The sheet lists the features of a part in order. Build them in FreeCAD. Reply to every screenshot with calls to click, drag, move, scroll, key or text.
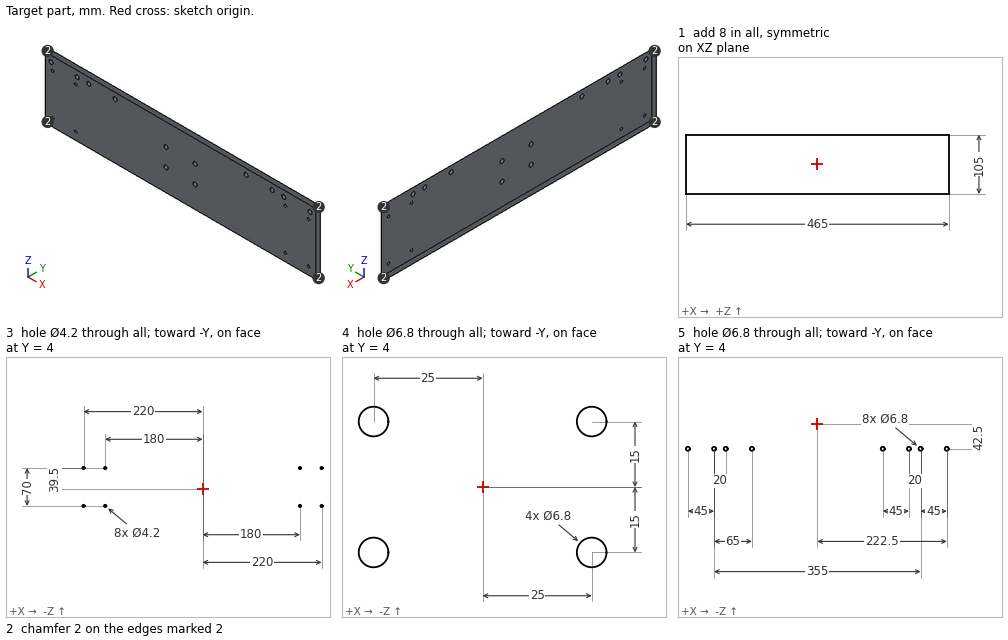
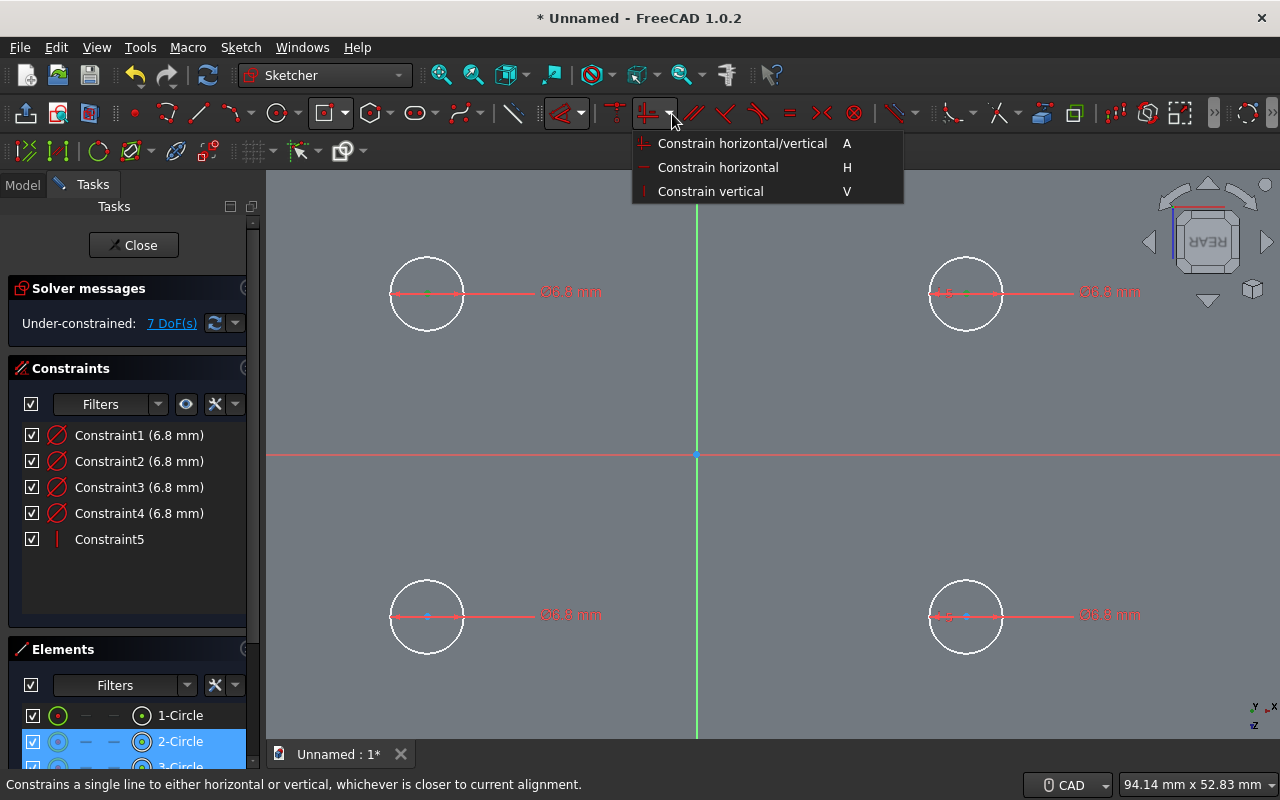
click(768, 167)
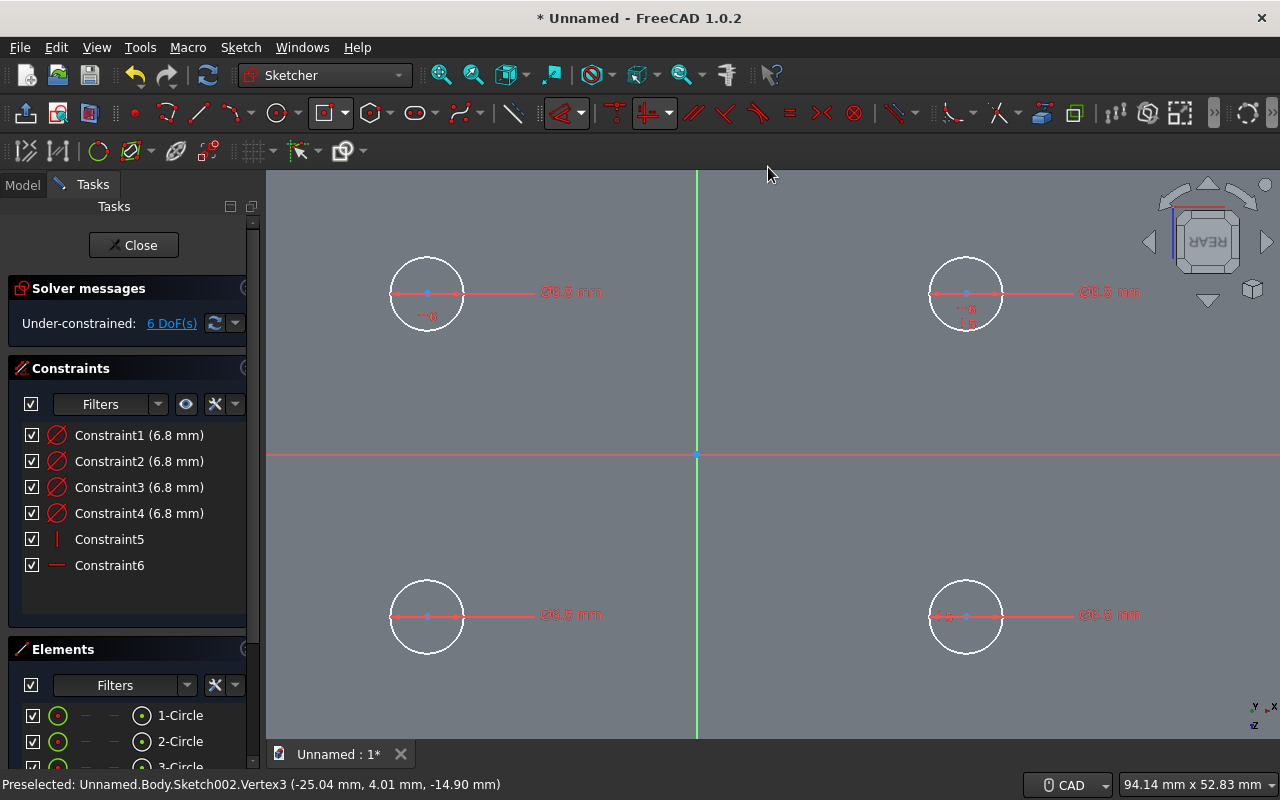
click(427, 294)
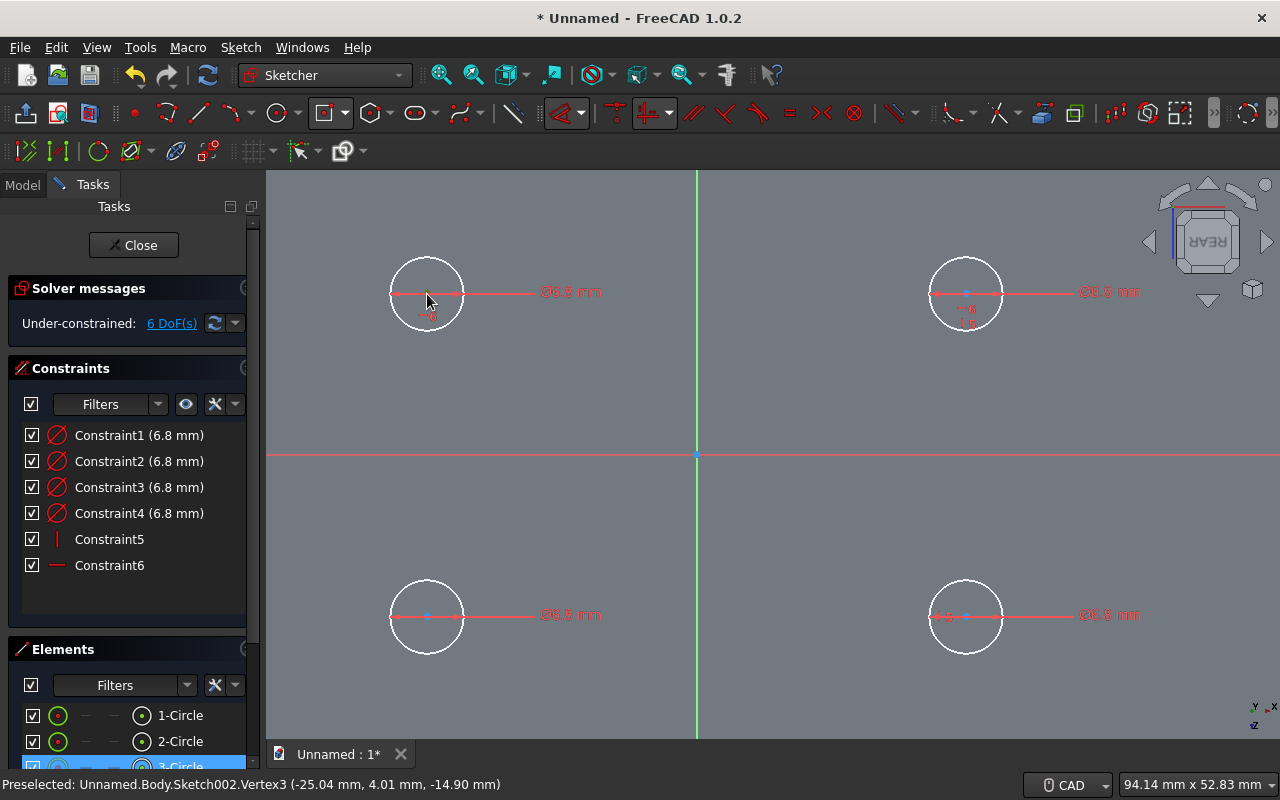
click(427, 617)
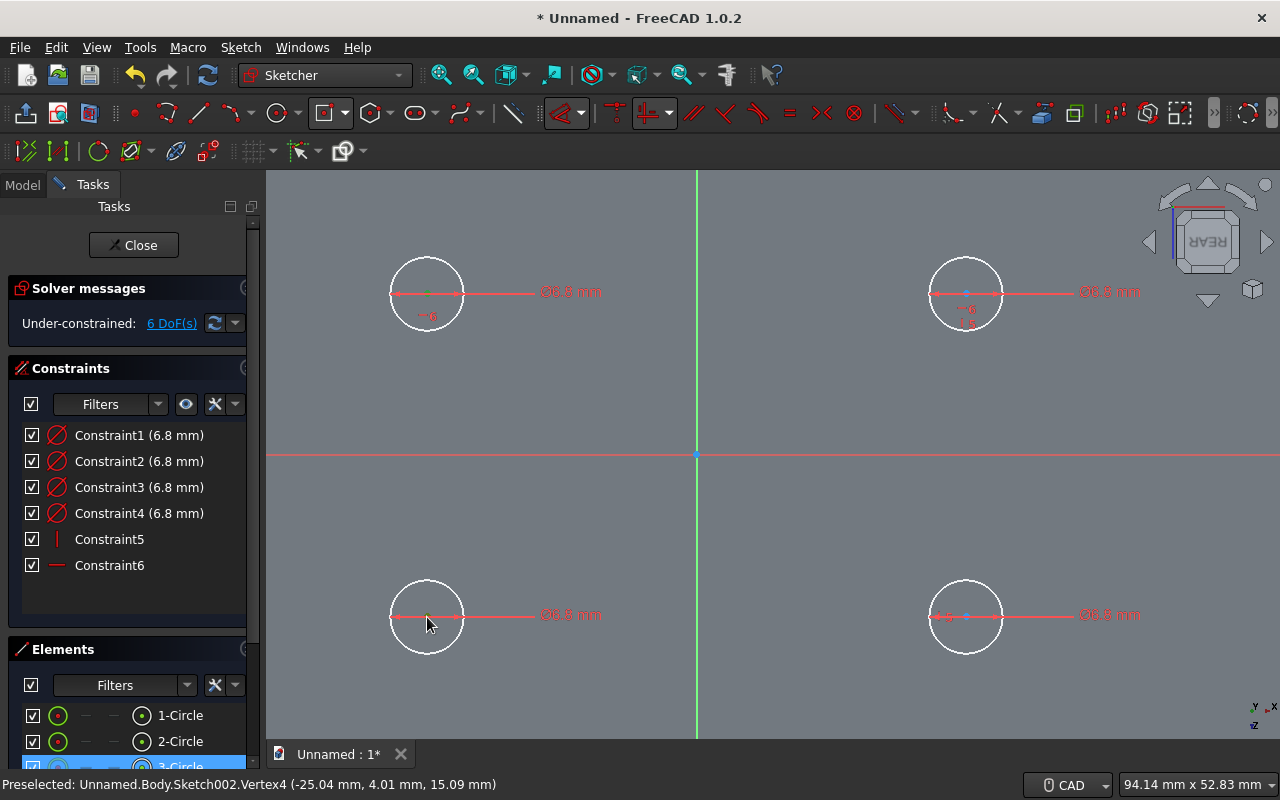
key(v)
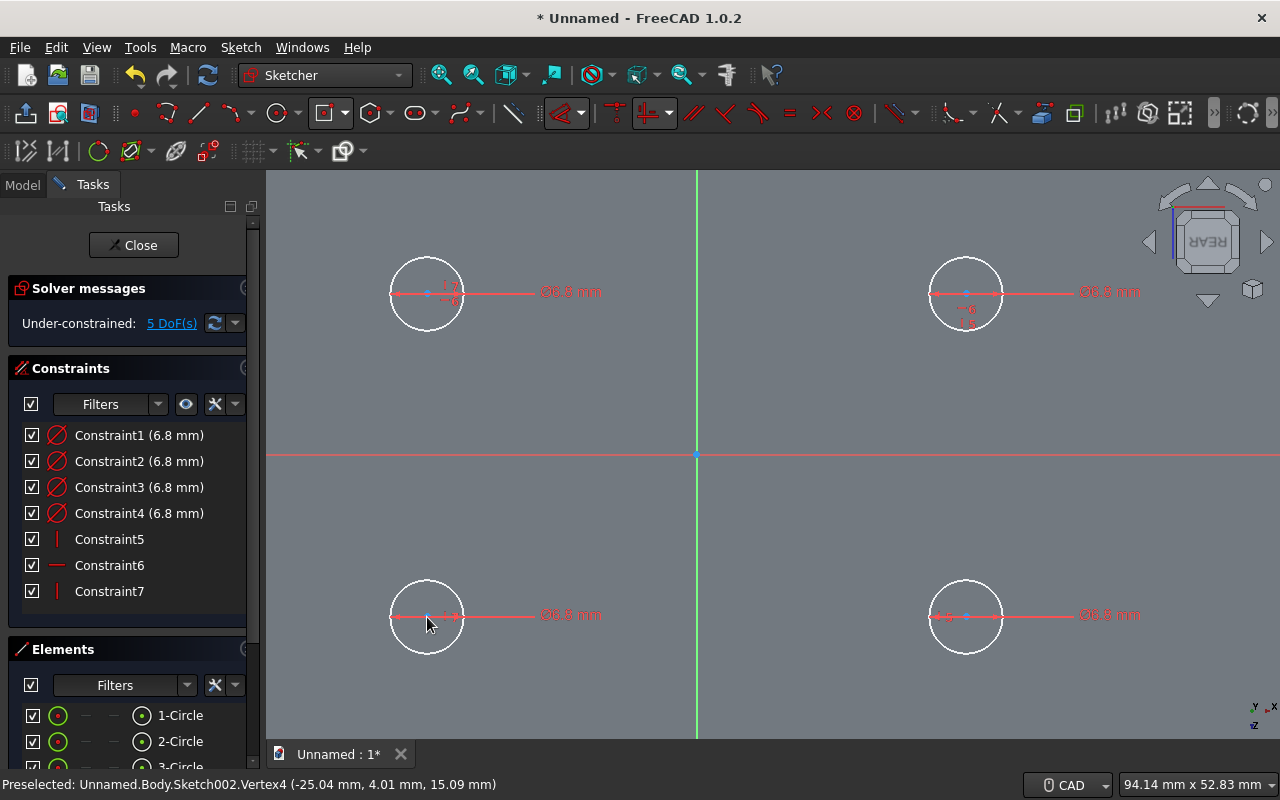
click(966, 617)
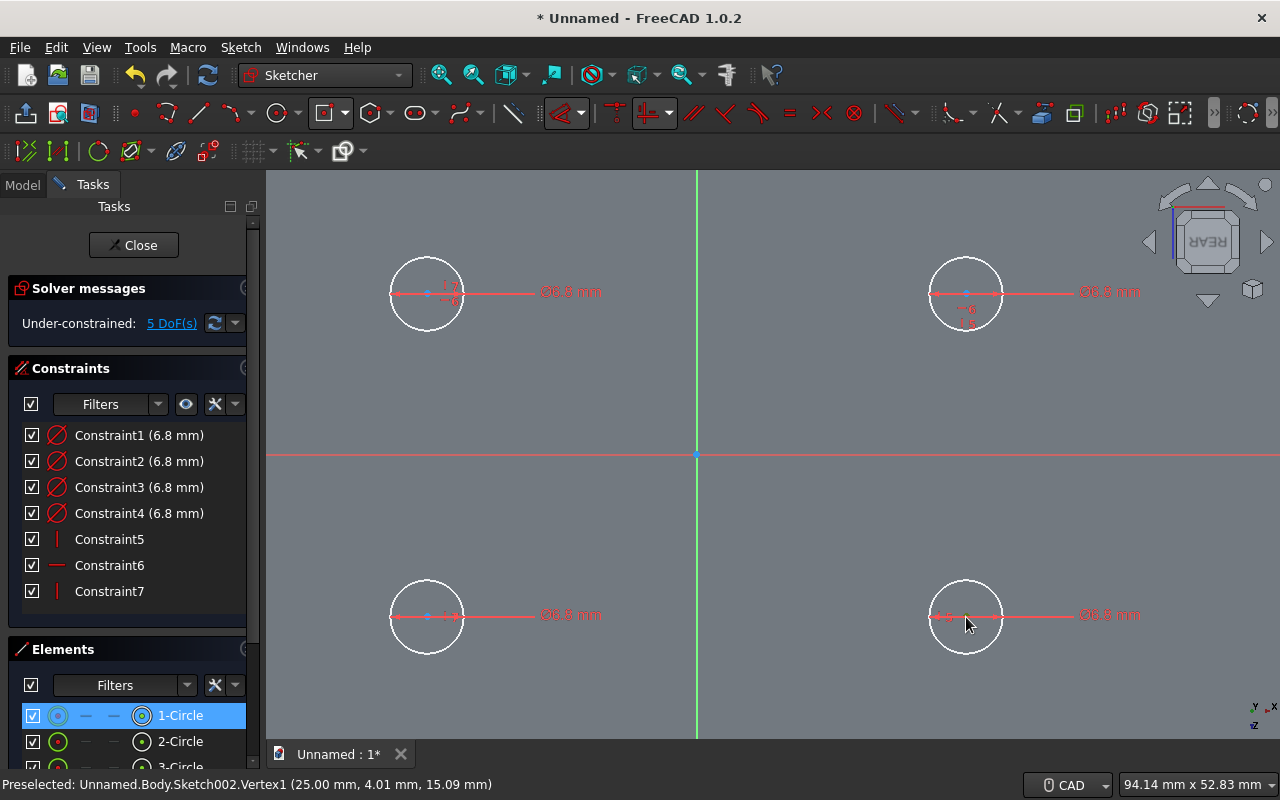
click(427, 617)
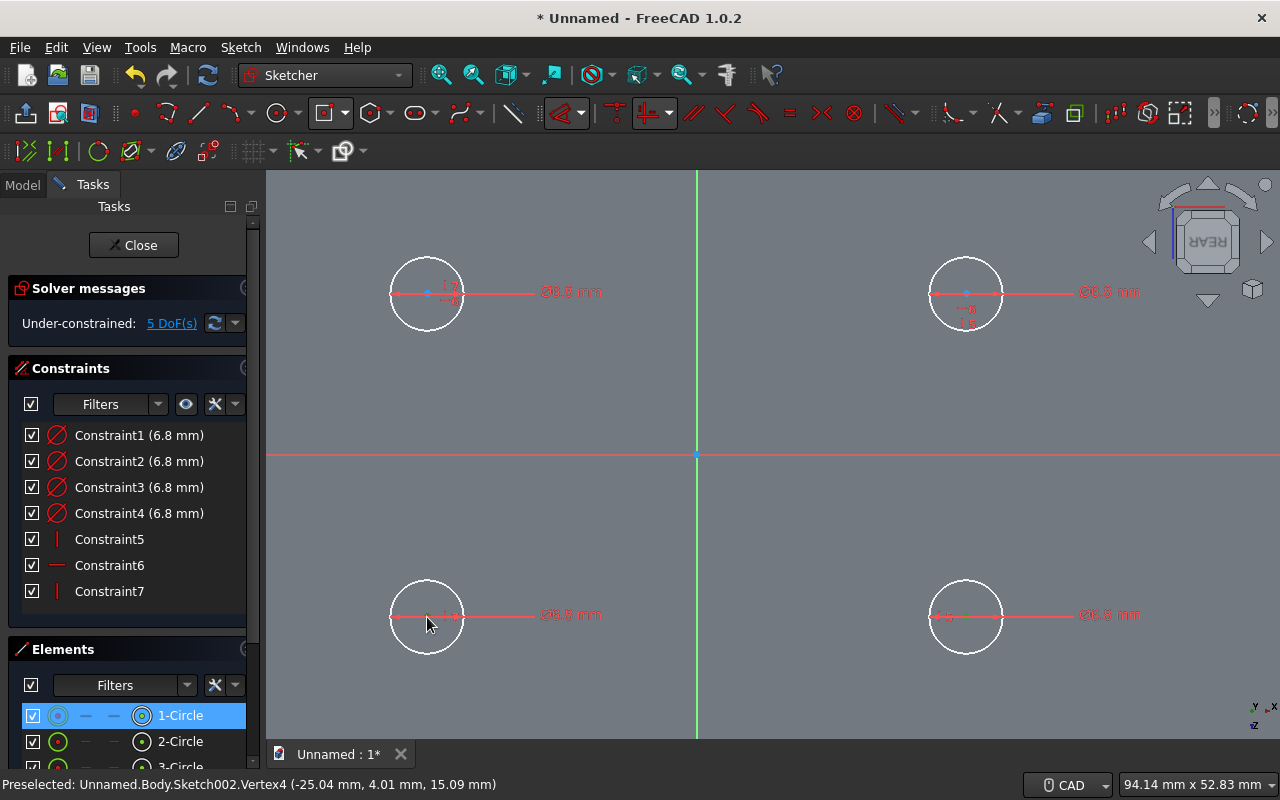
key(h)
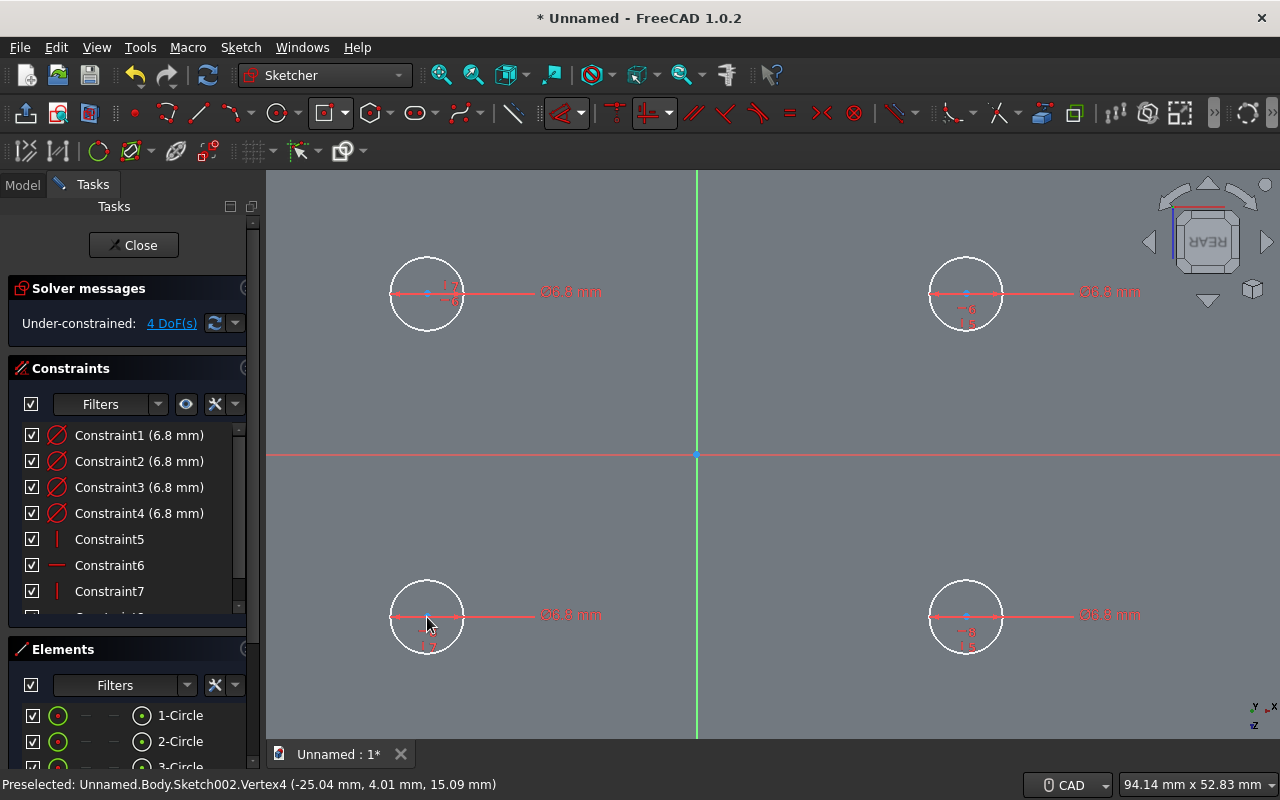
click(966, 617)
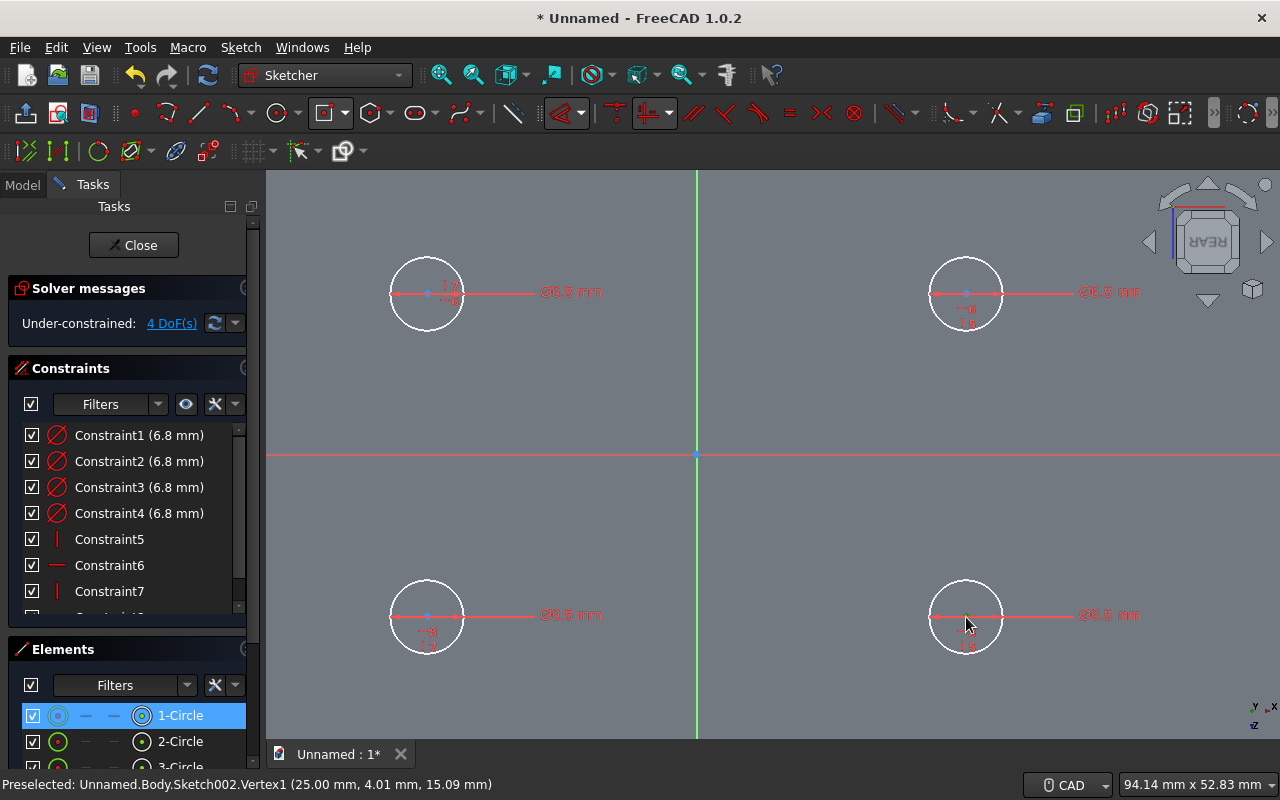
click(584, 114)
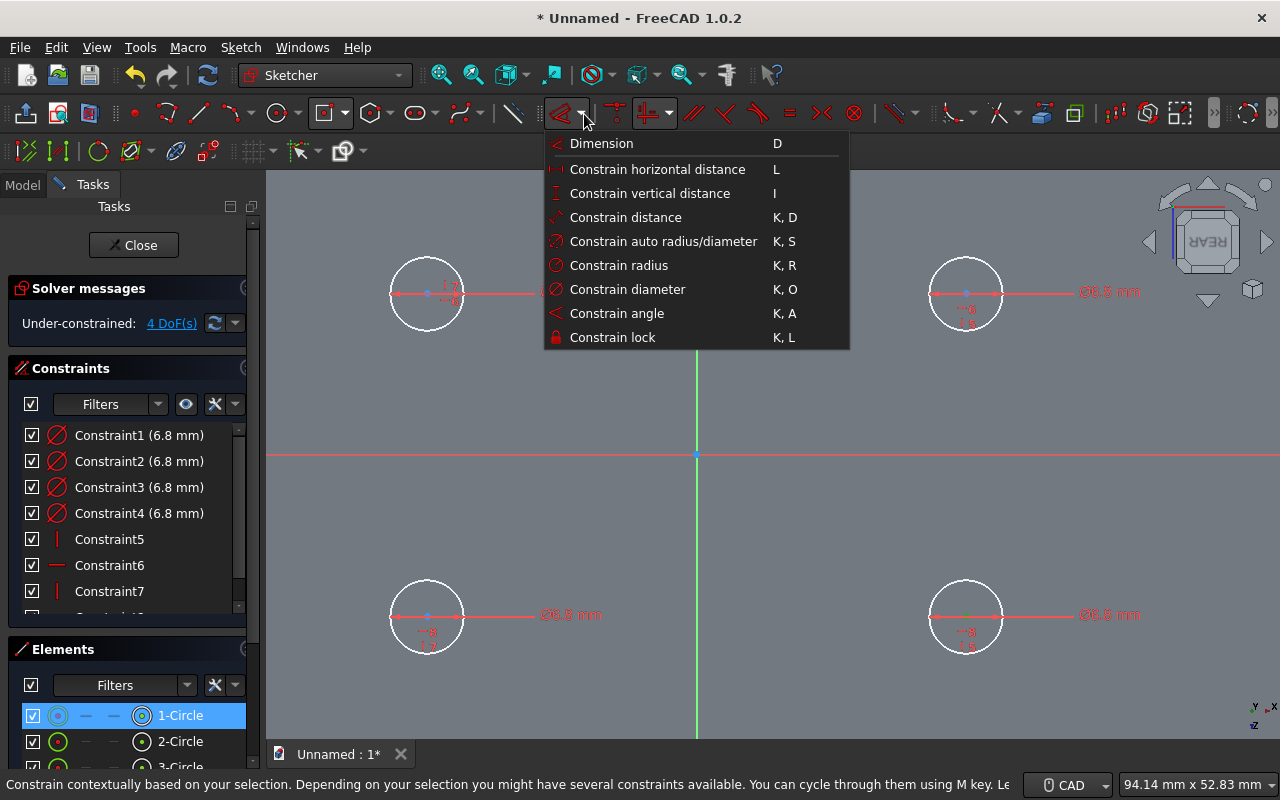
click(697, 169)